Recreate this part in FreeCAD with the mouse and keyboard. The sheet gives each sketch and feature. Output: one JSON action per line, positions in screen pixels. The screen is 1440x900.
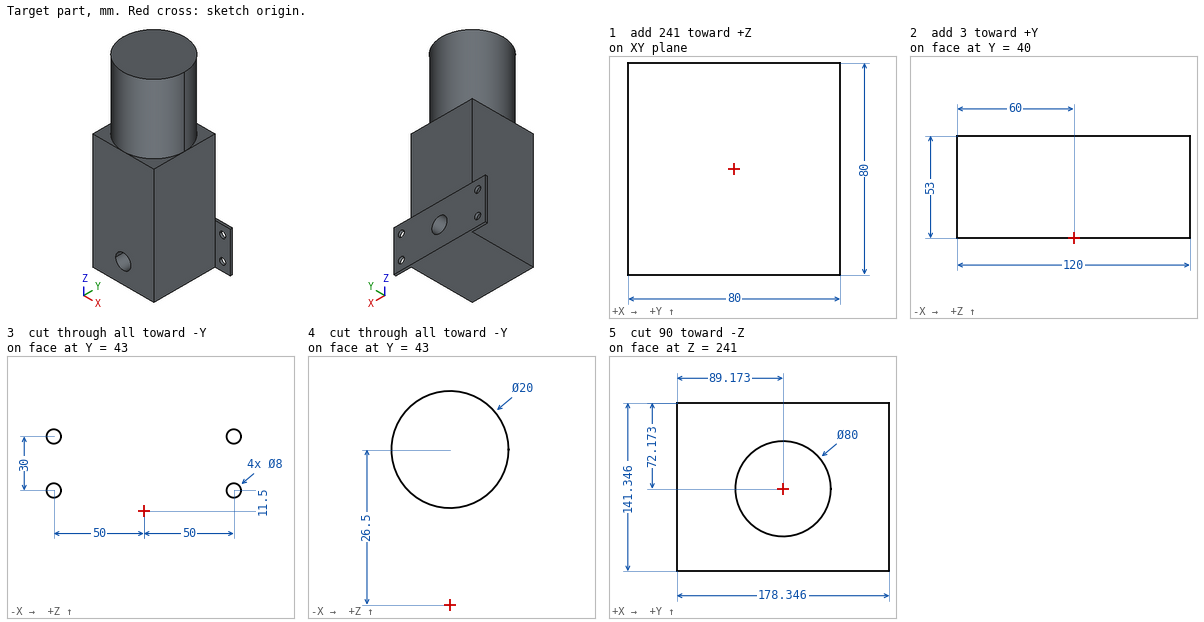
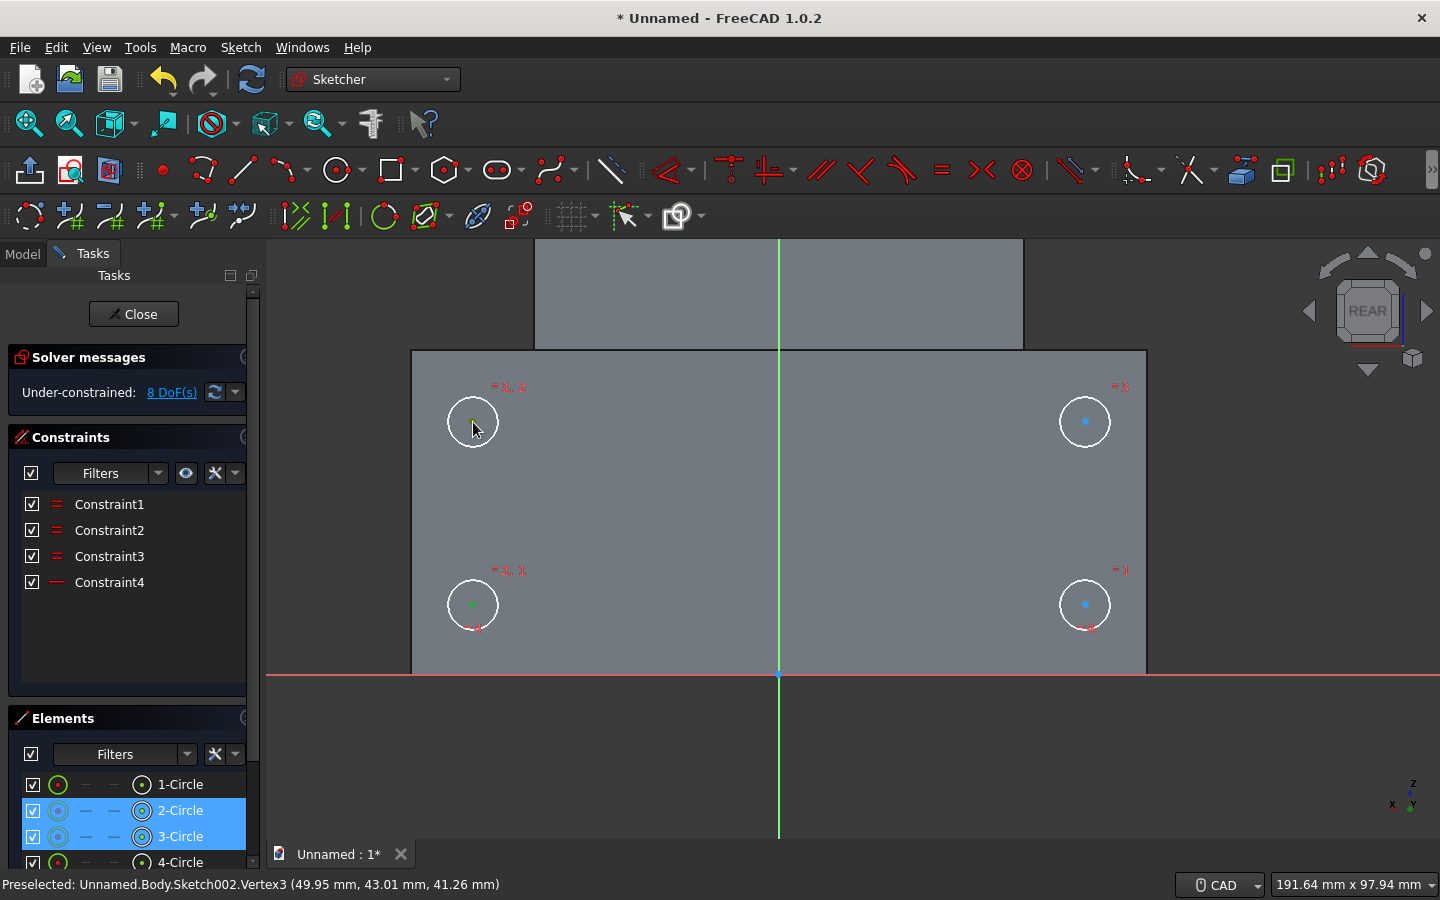
{"action": "left_click", "coordinate": [796, 170]}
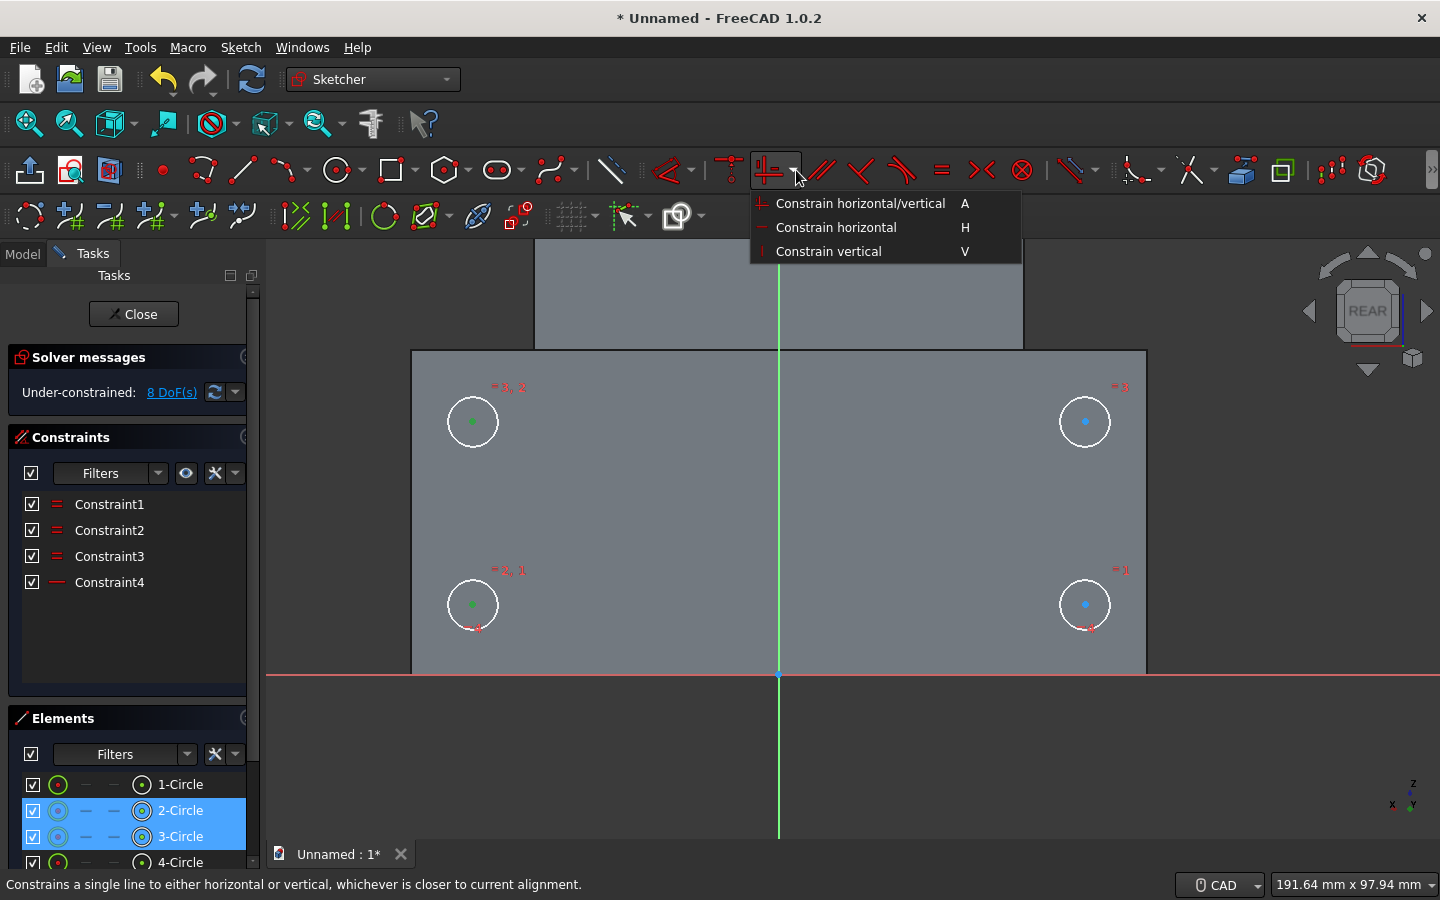
{"action": "left_click", "coordinate": [886, 251]}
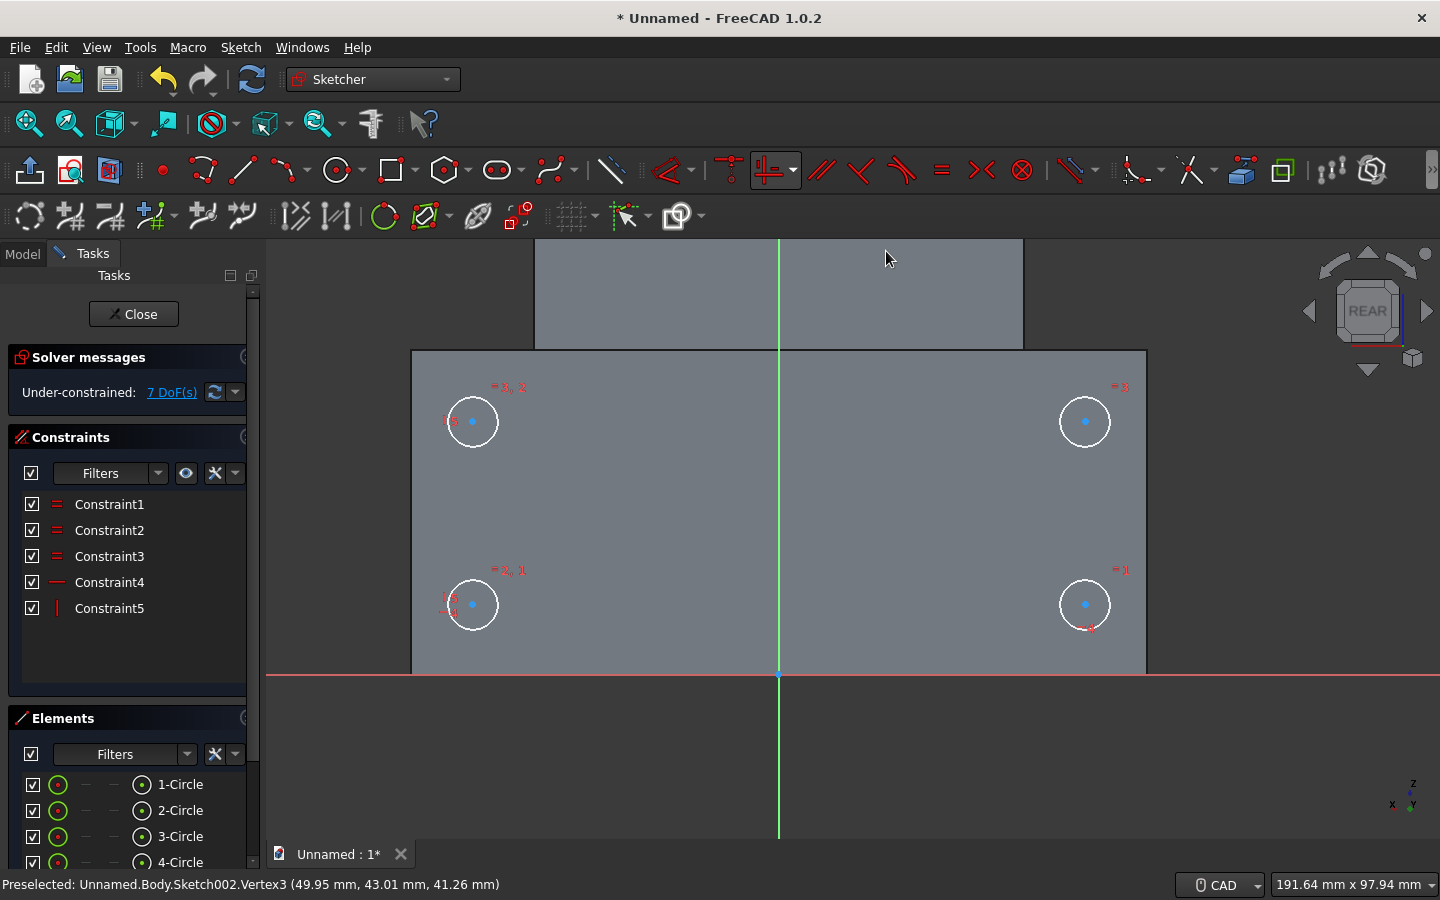
{"action": "left_click", "coordinate": [1085, 605]}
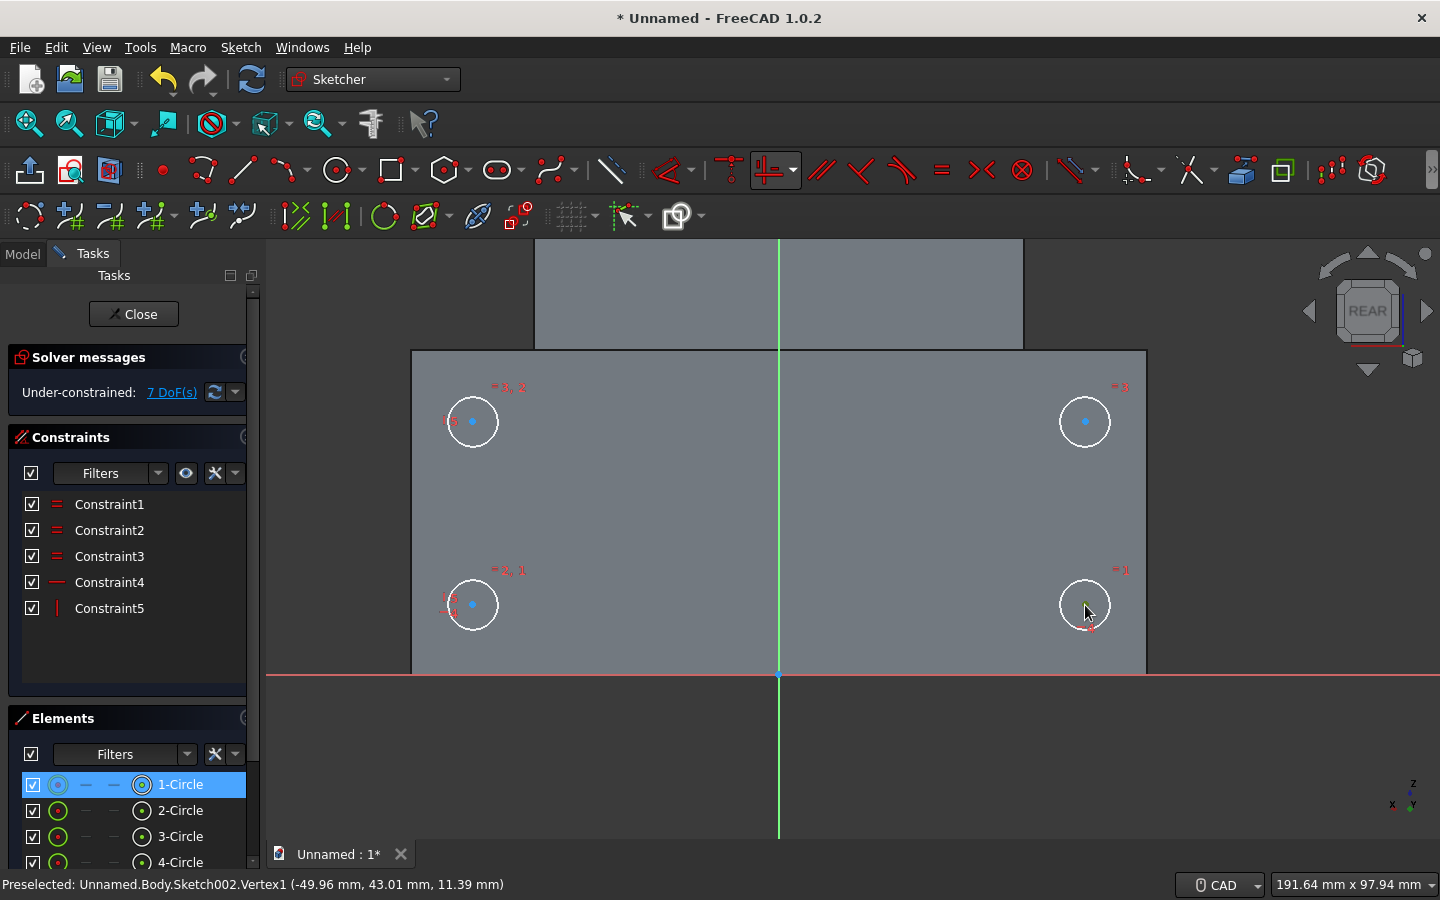
{"action": "left_click", "coordinate": [1085, 422]}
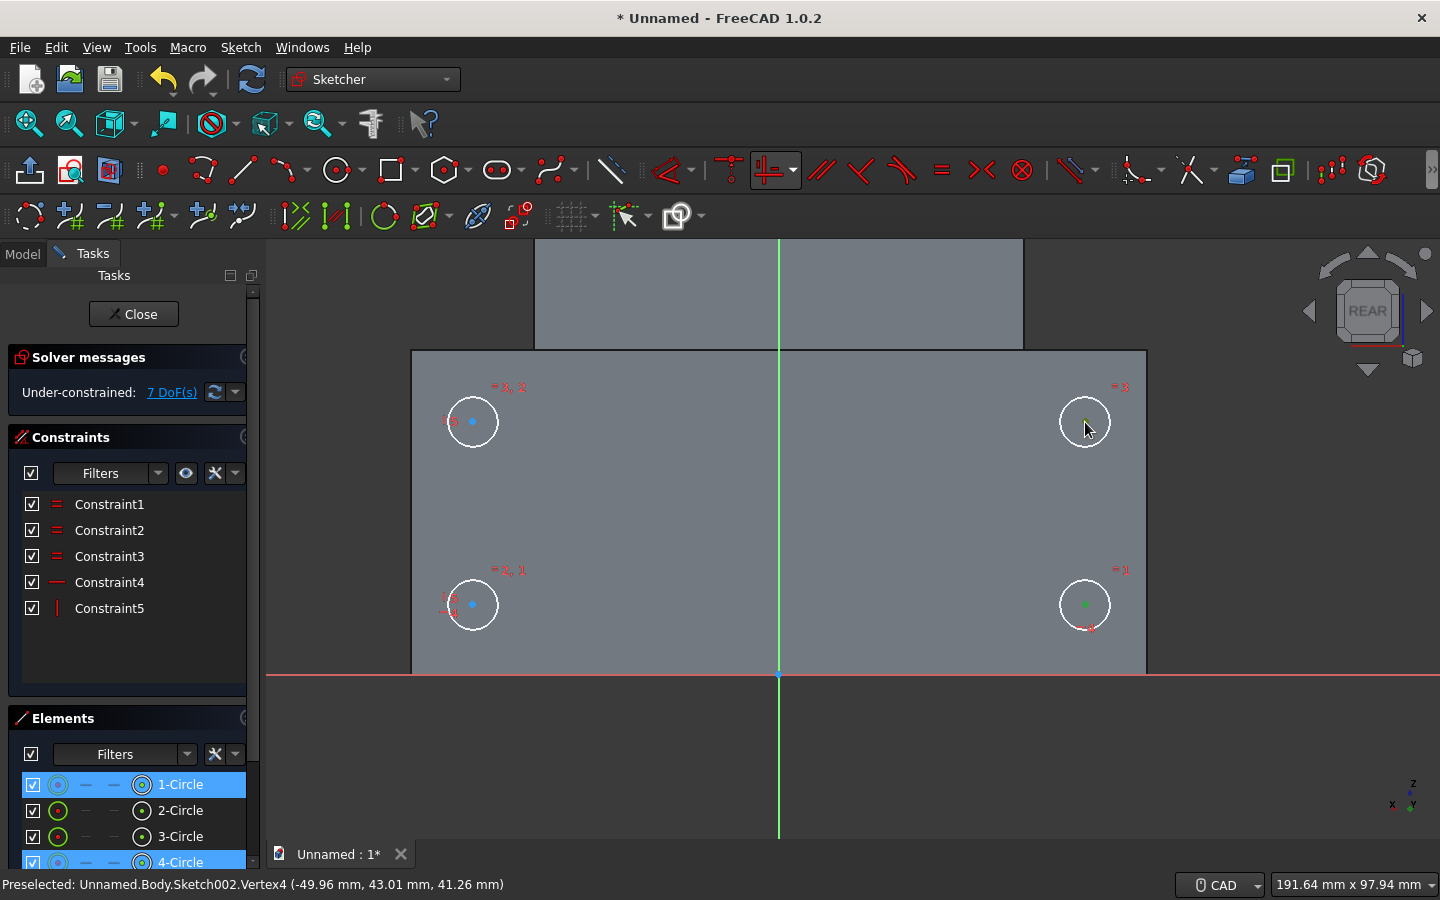
{"action": "key", "text": "v"}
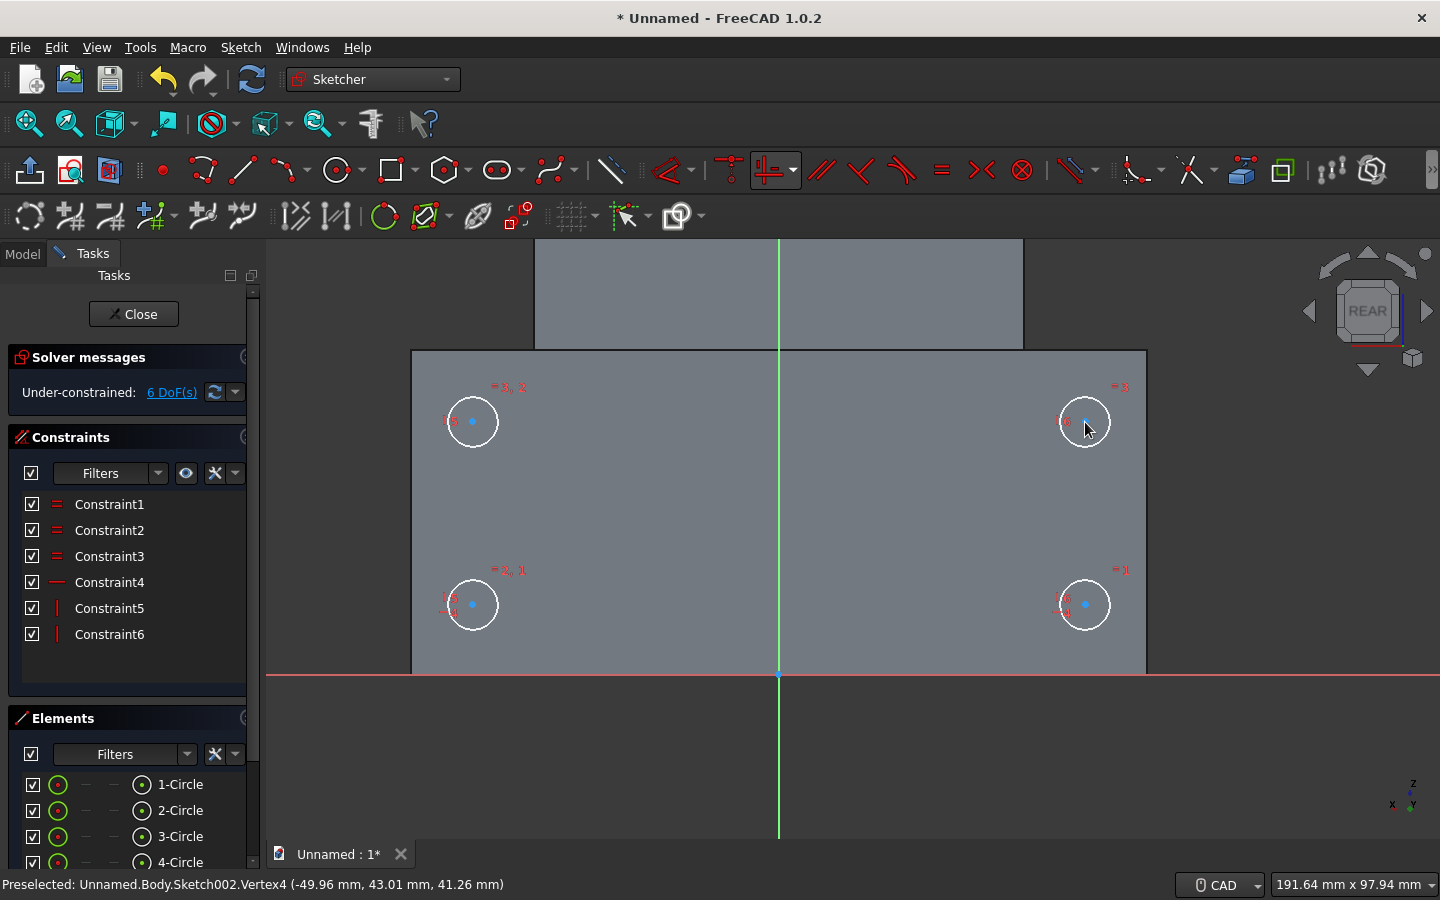
{"action": "left_click", "coordinate": [473, 422]}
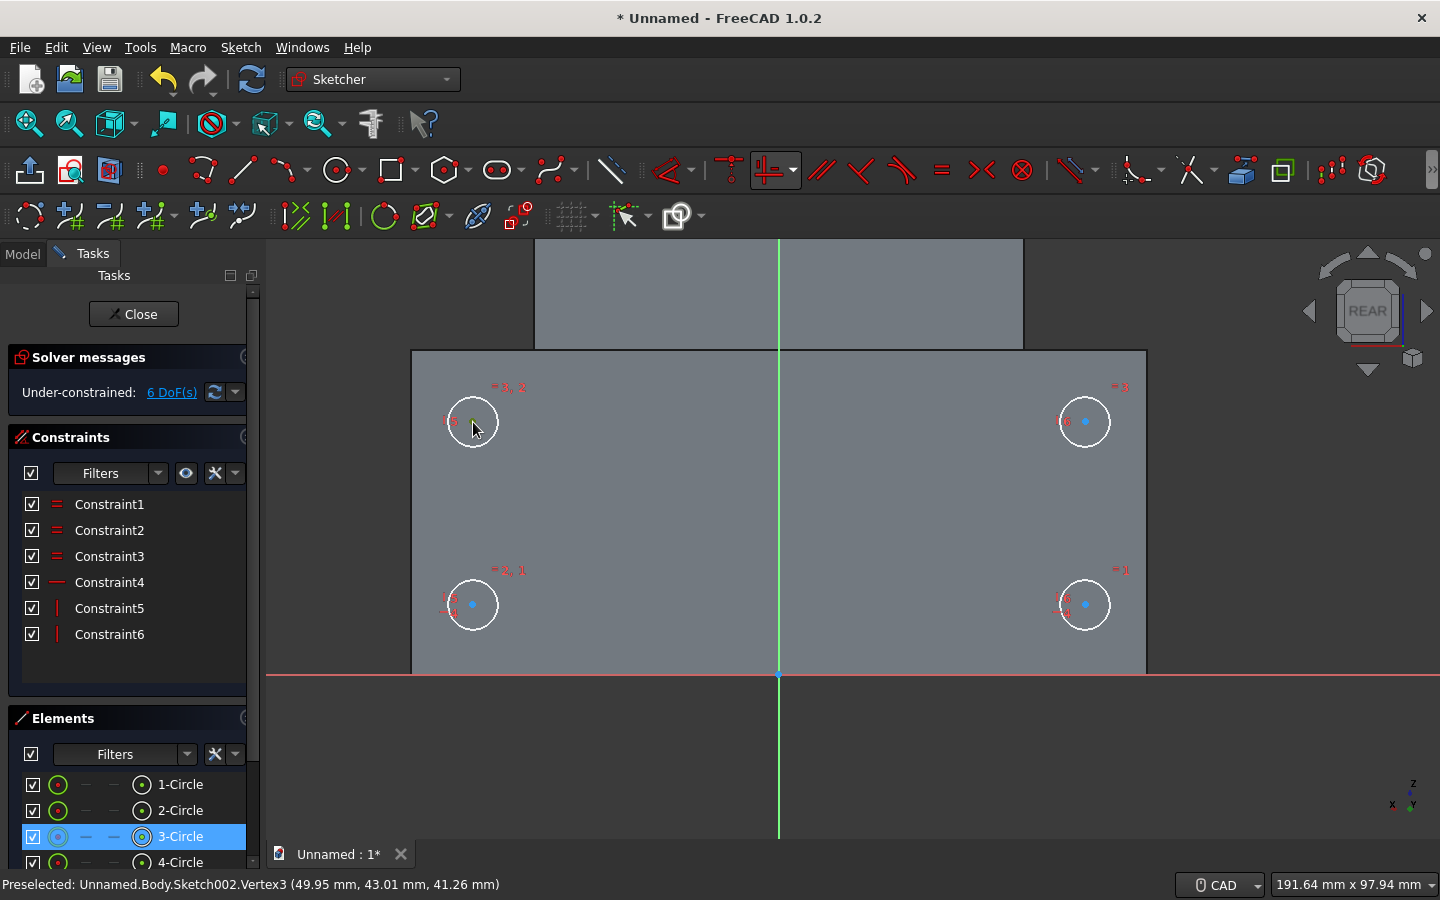
{"action": "left_click", "coordinate": [1085, 422]}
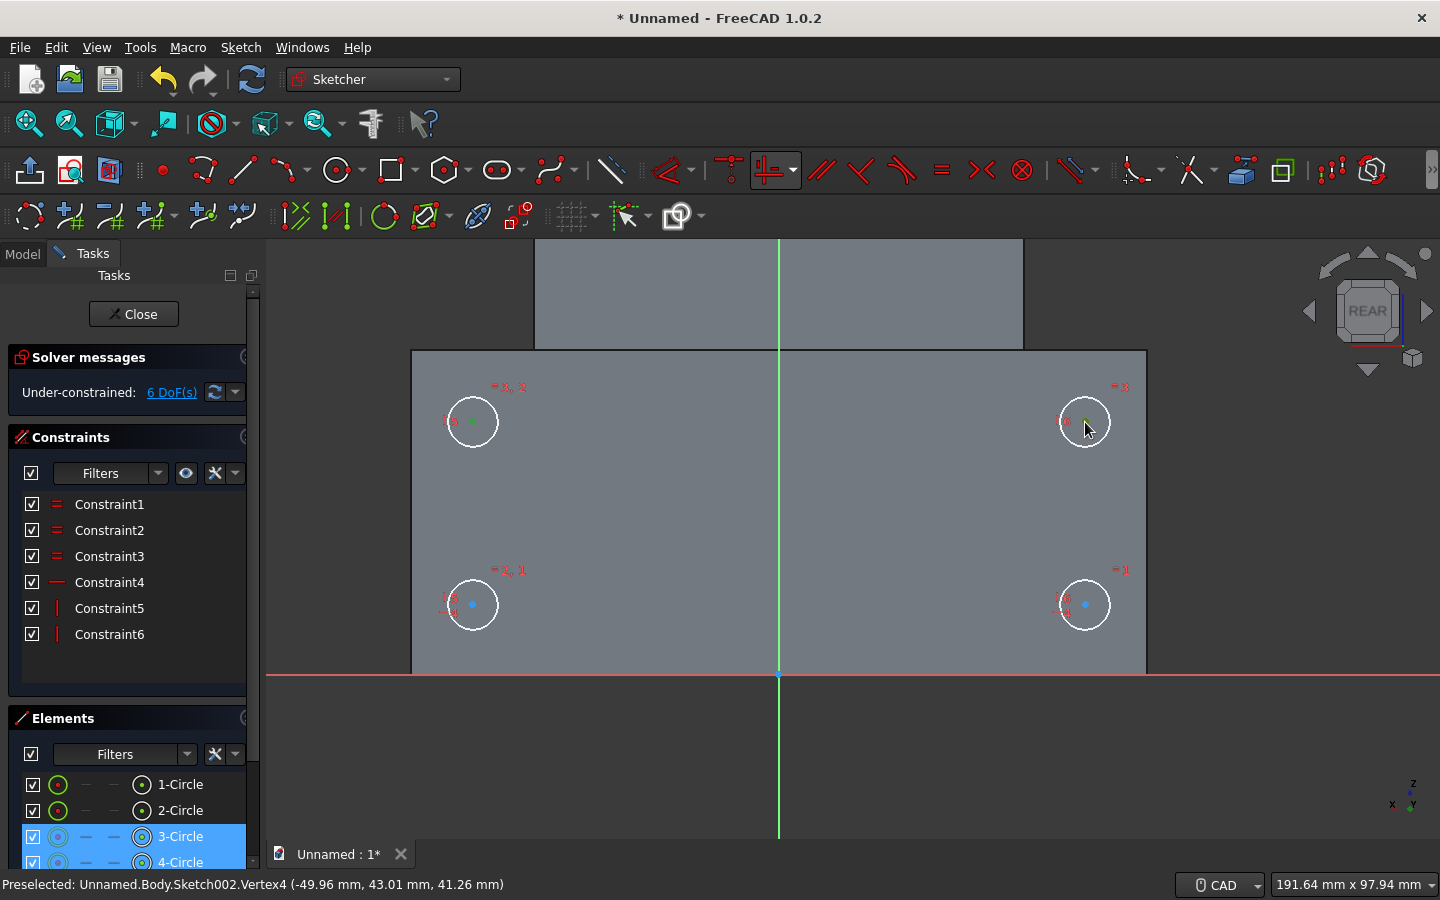
{"action": "key", "text": "h"}